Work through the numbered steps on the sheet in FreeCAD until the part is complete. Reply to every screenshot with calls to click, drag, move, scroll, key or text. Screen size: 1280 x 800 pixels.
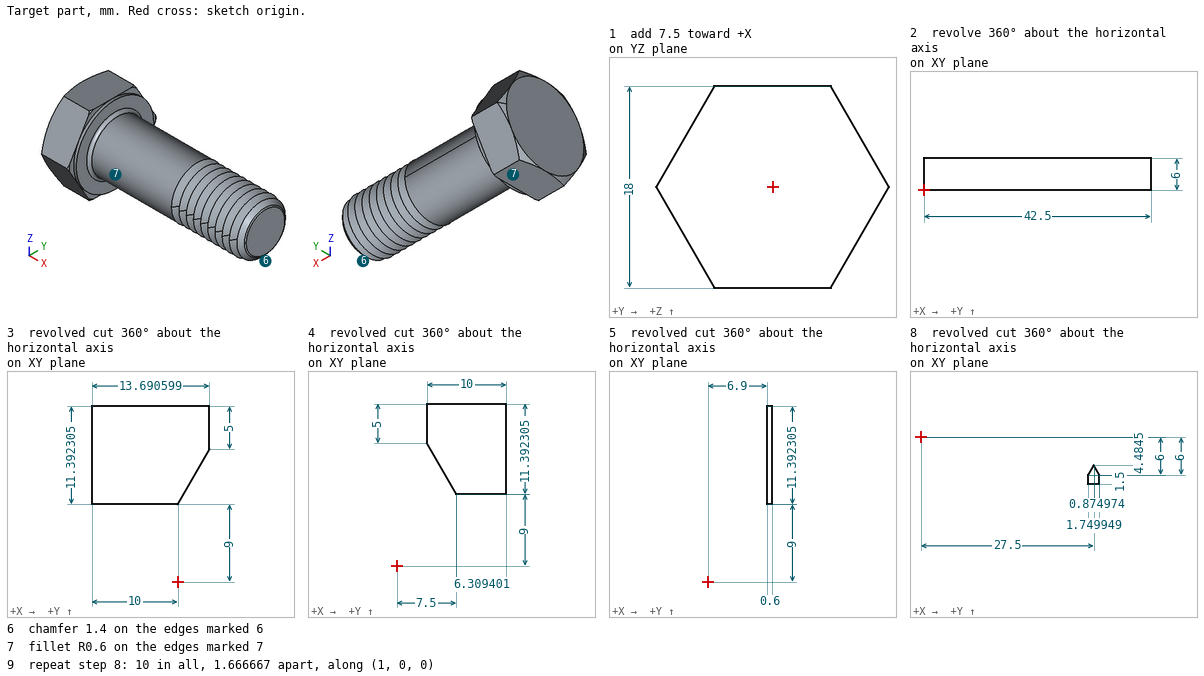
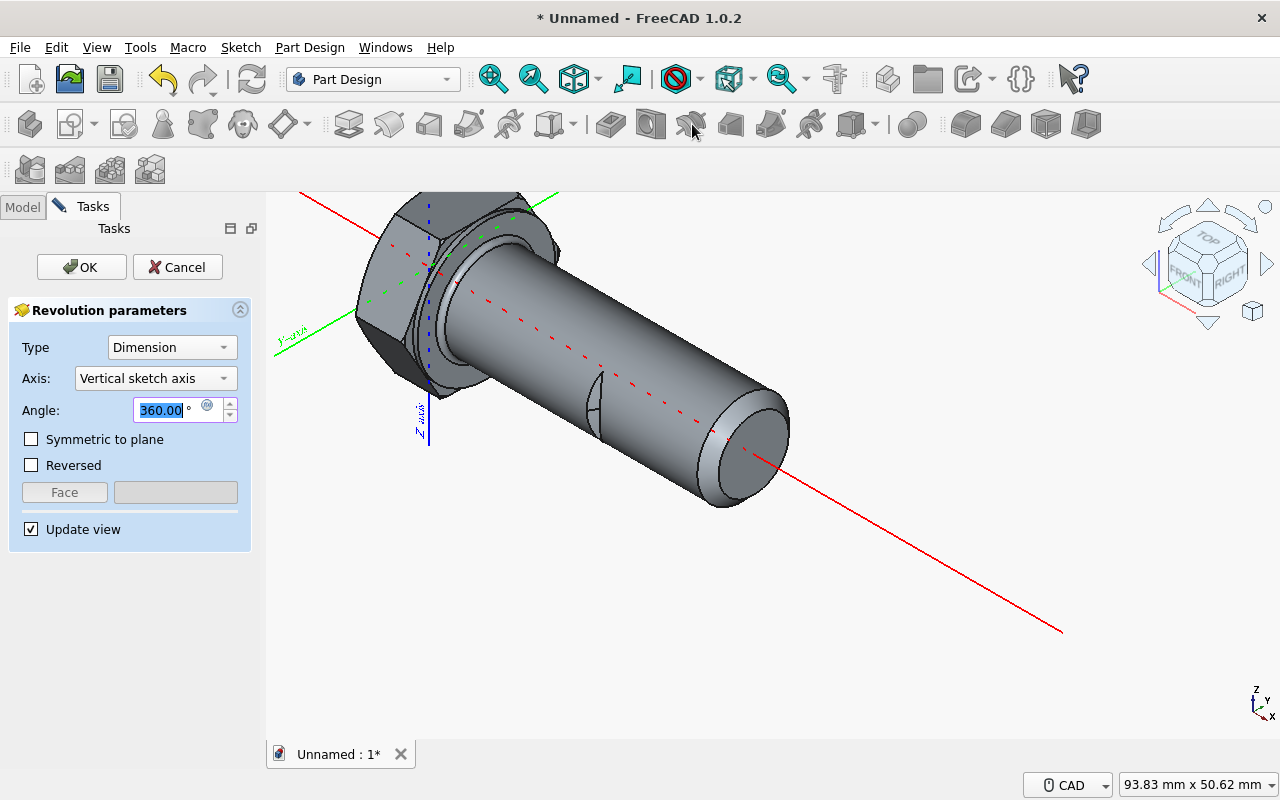
click(156, 378)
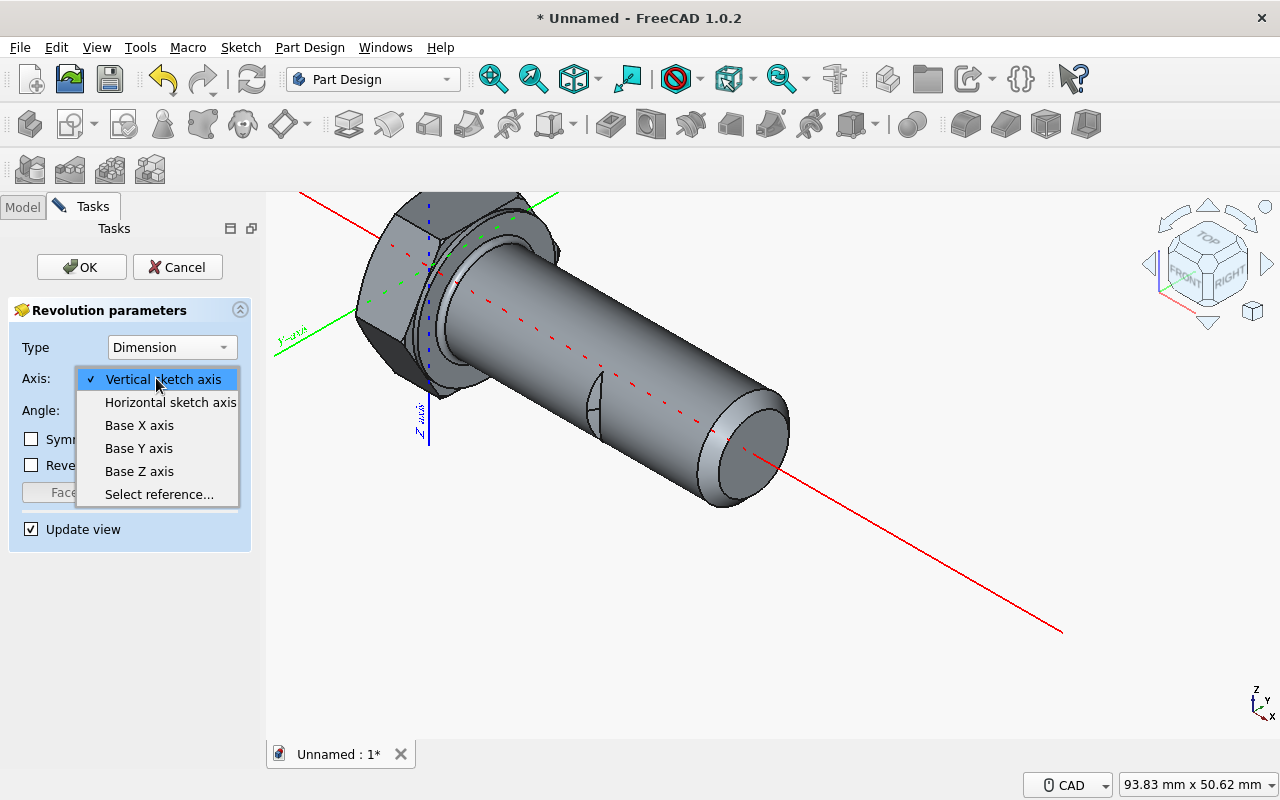
click(156, 402)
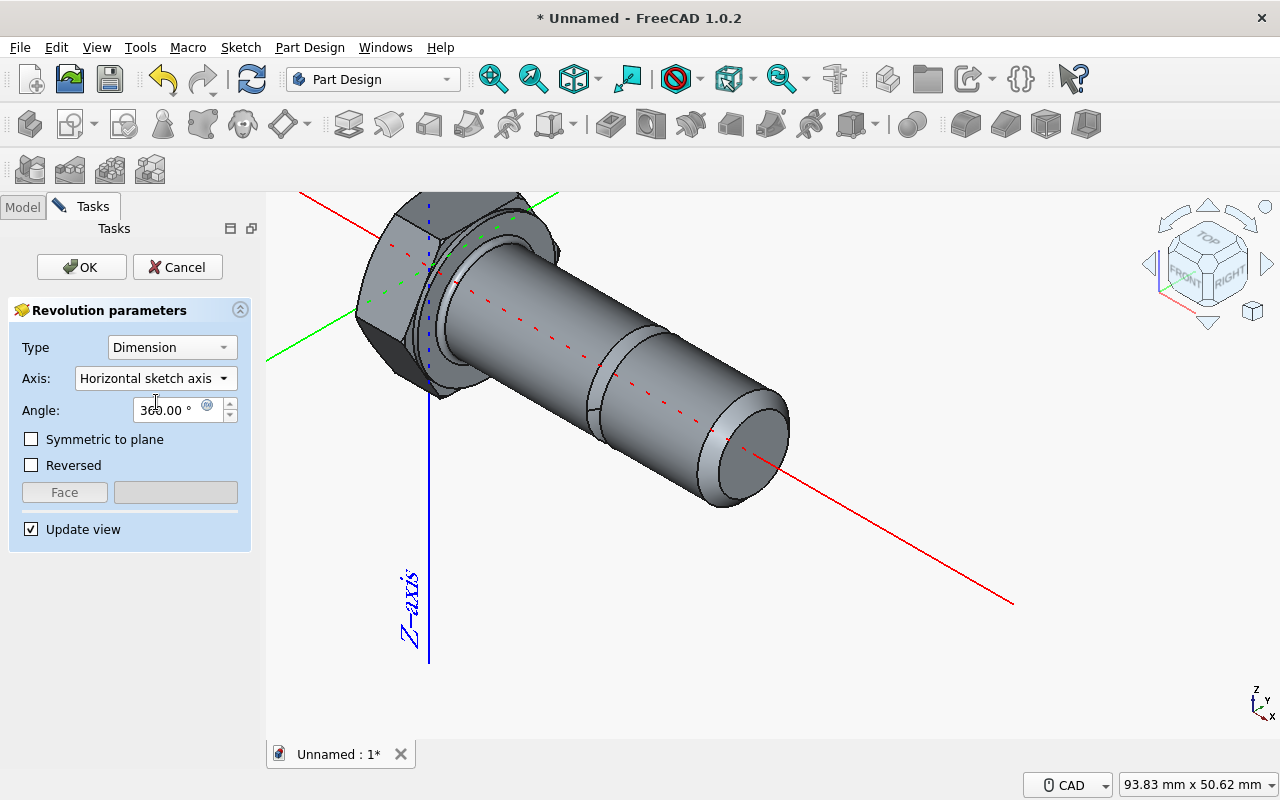
click(82, 267)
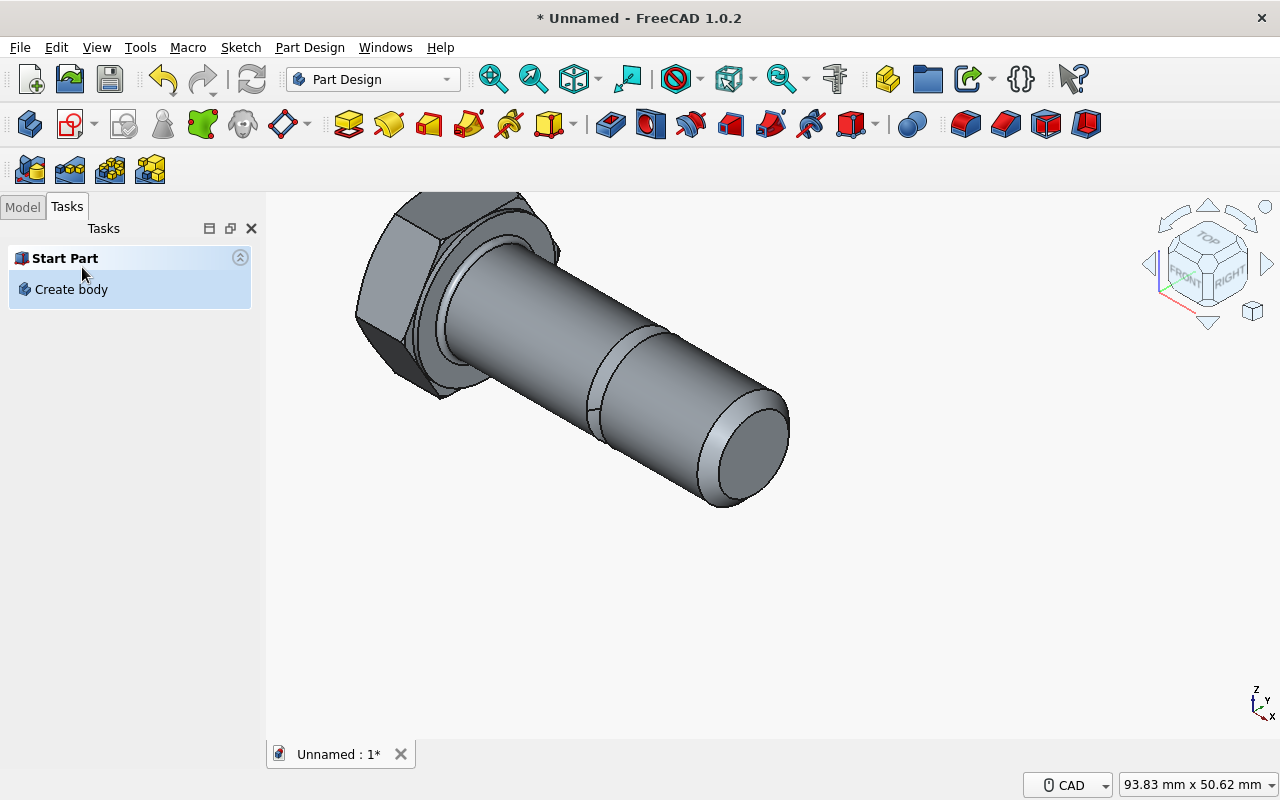
key(v)
key(f)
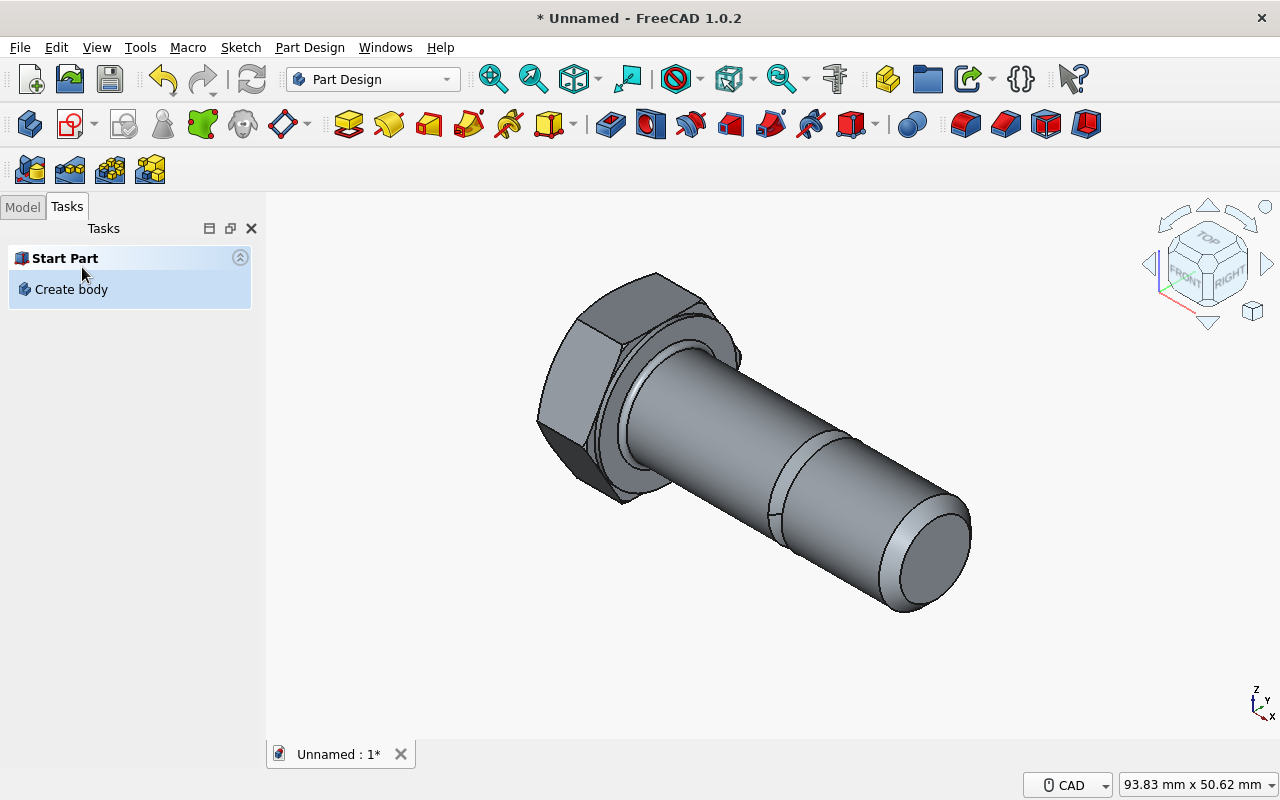
click(23, 206)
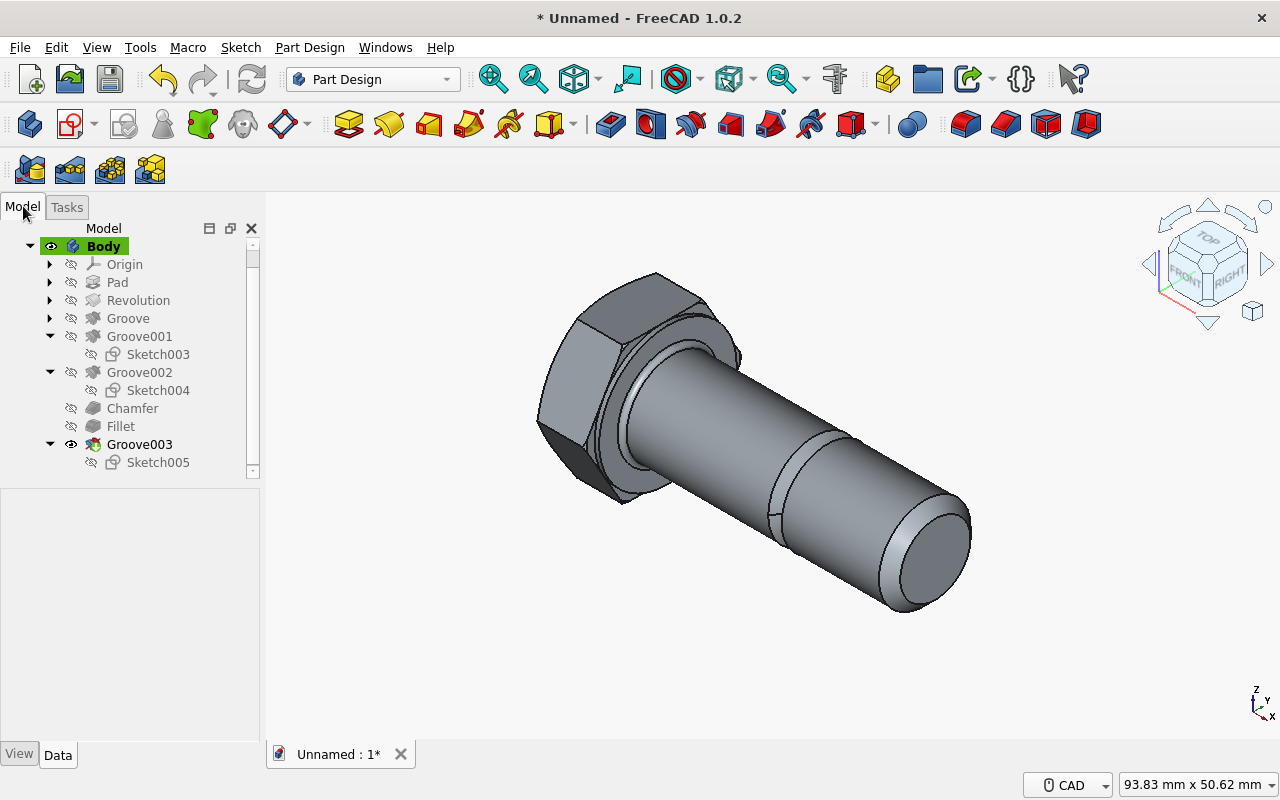
click(116, 444)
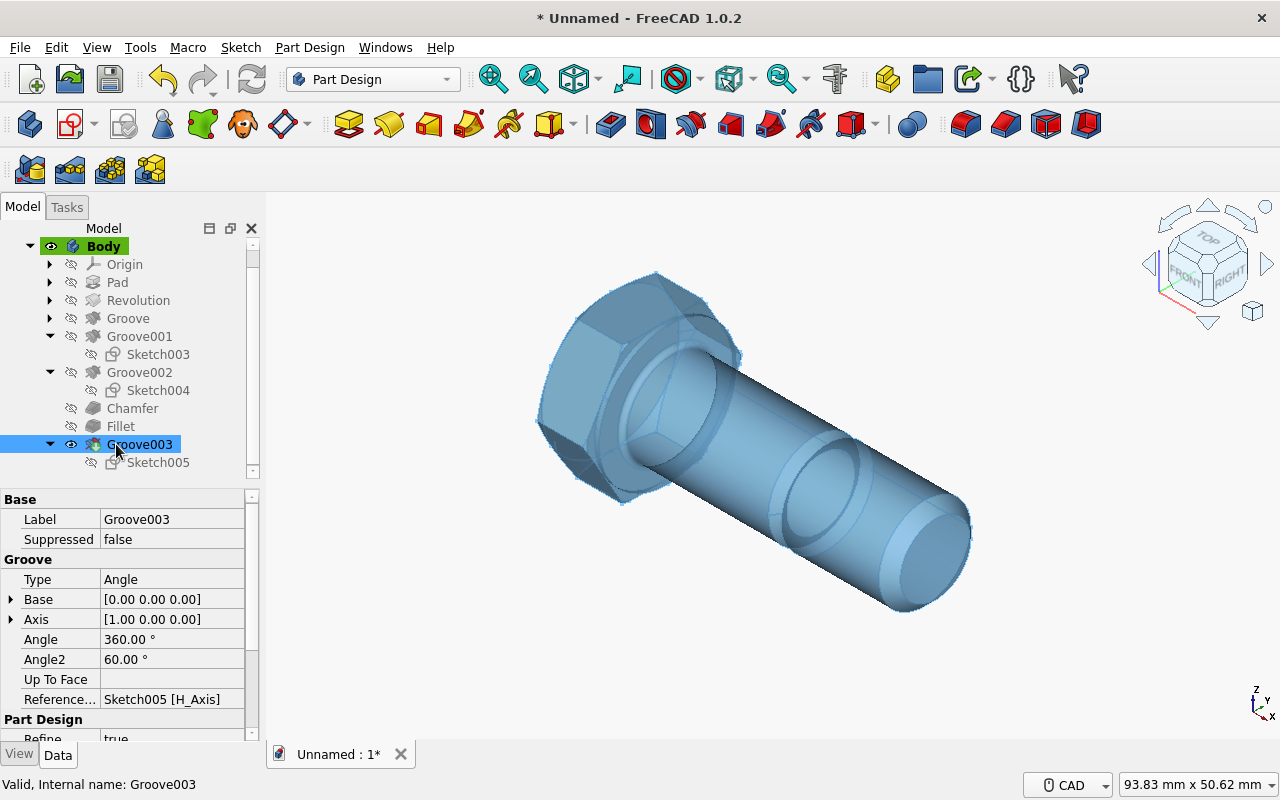
click(70, 170)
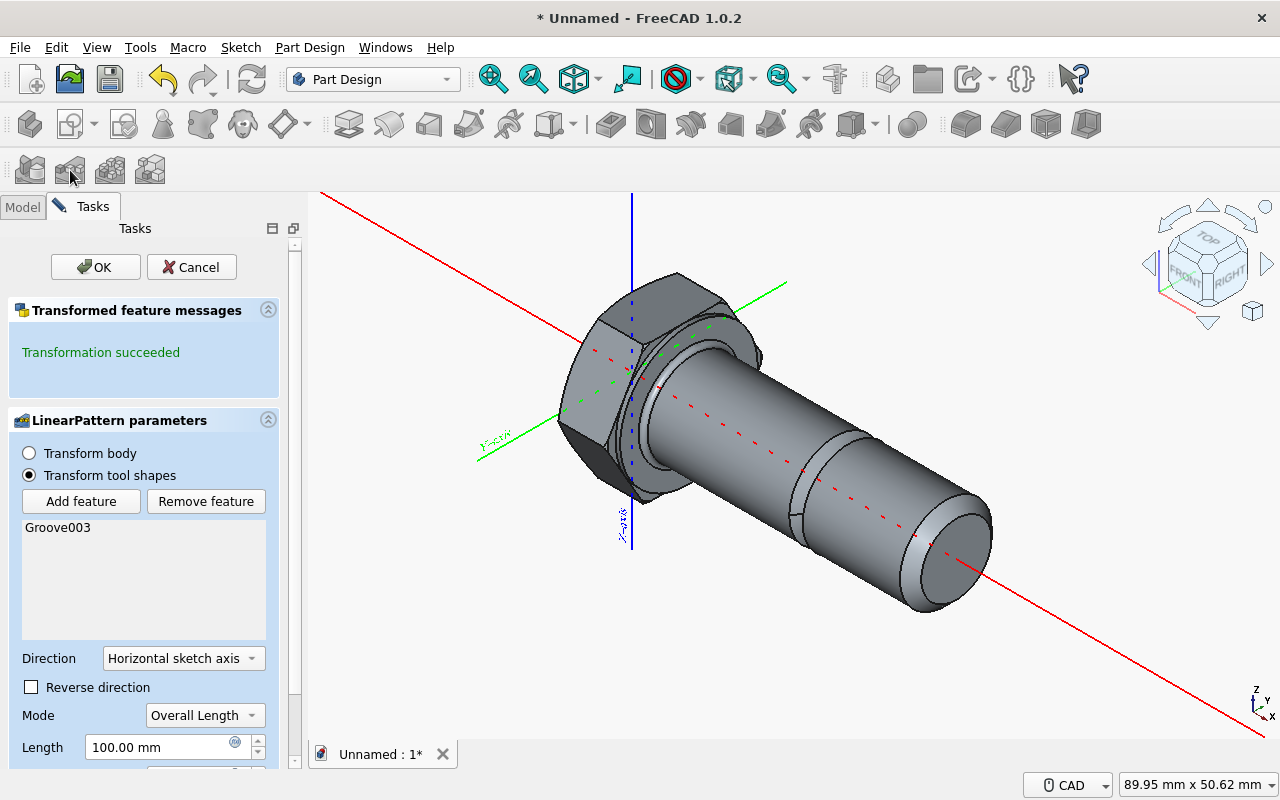
click(184, 658)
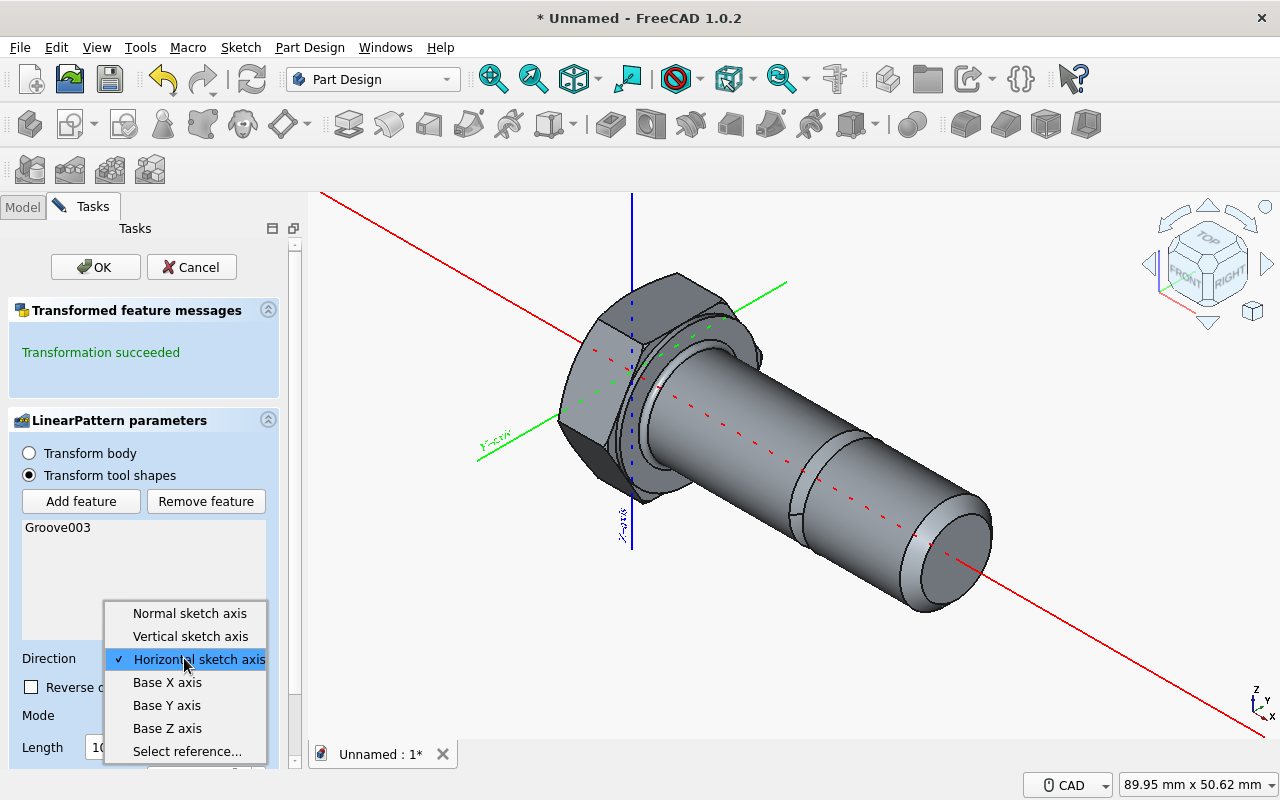
click(184, 682)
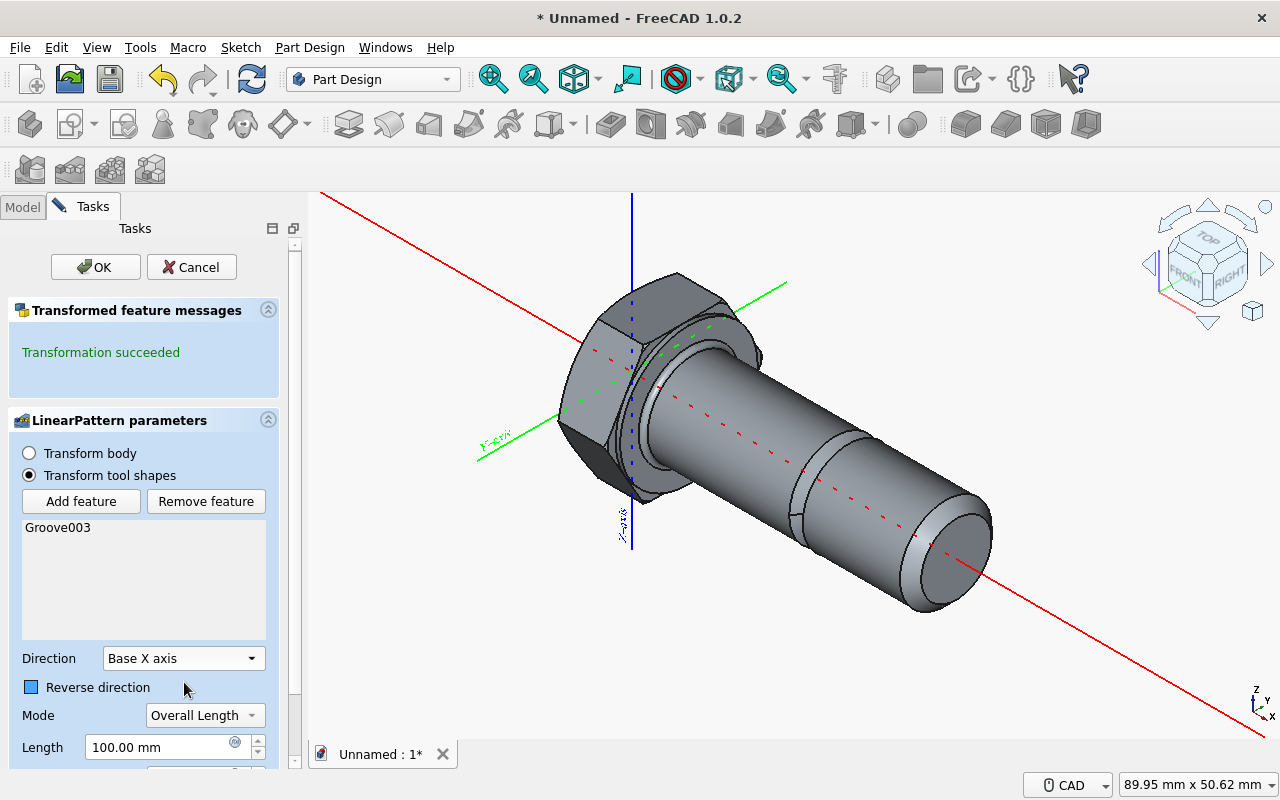
click(206, 716)